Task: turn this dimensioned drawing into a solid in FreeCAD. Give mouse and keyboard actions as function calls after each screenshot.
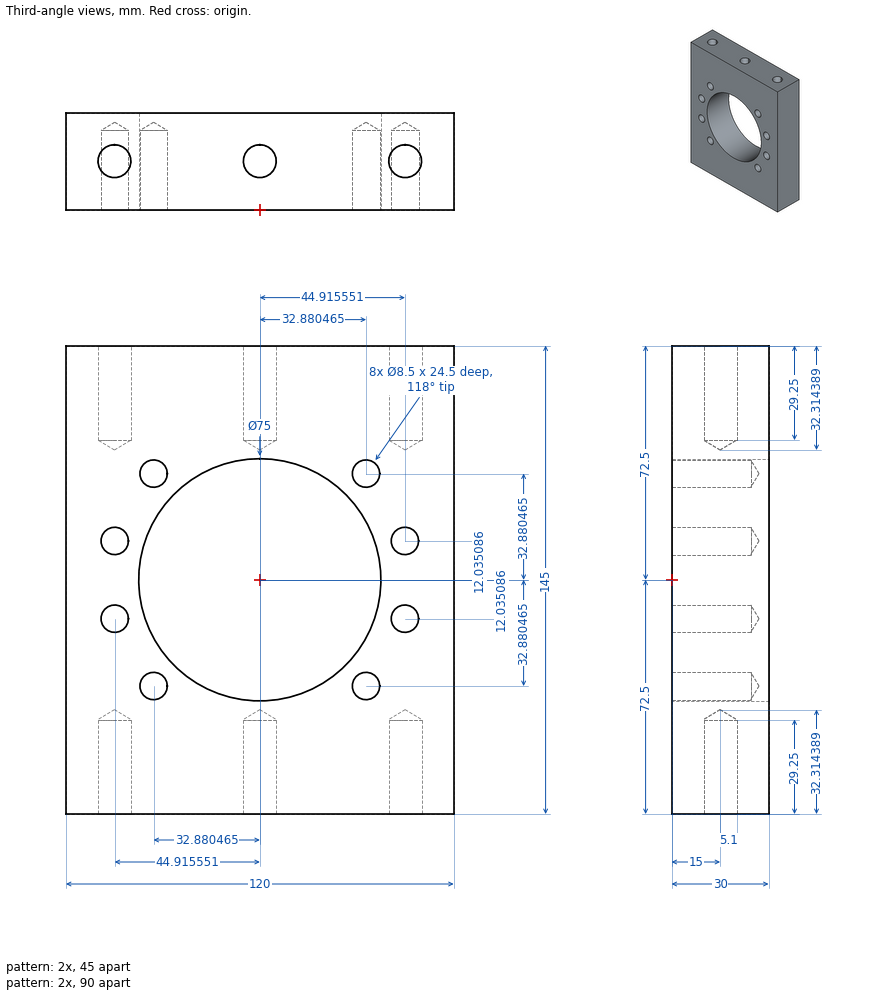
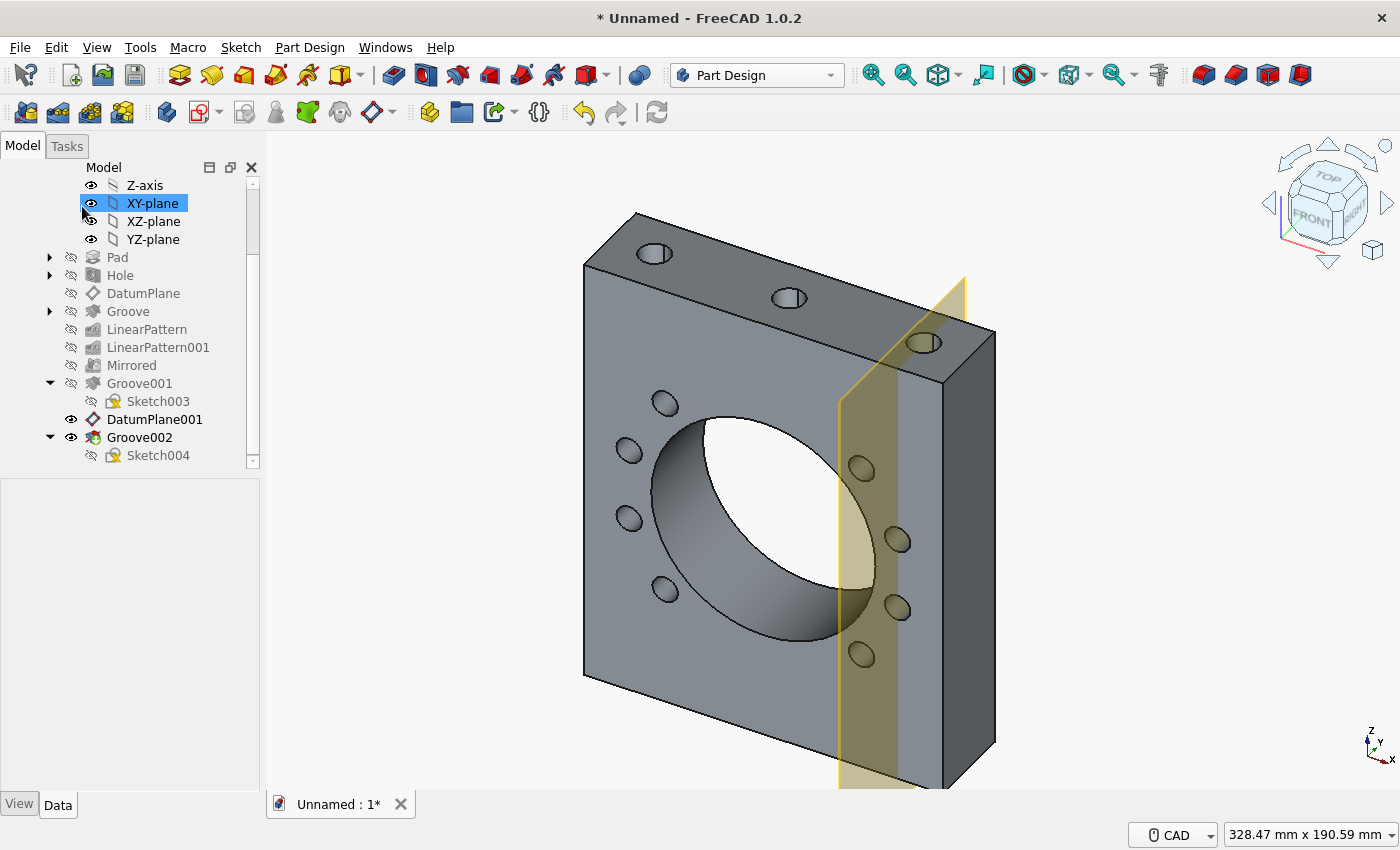
click(116, 419)
key(space)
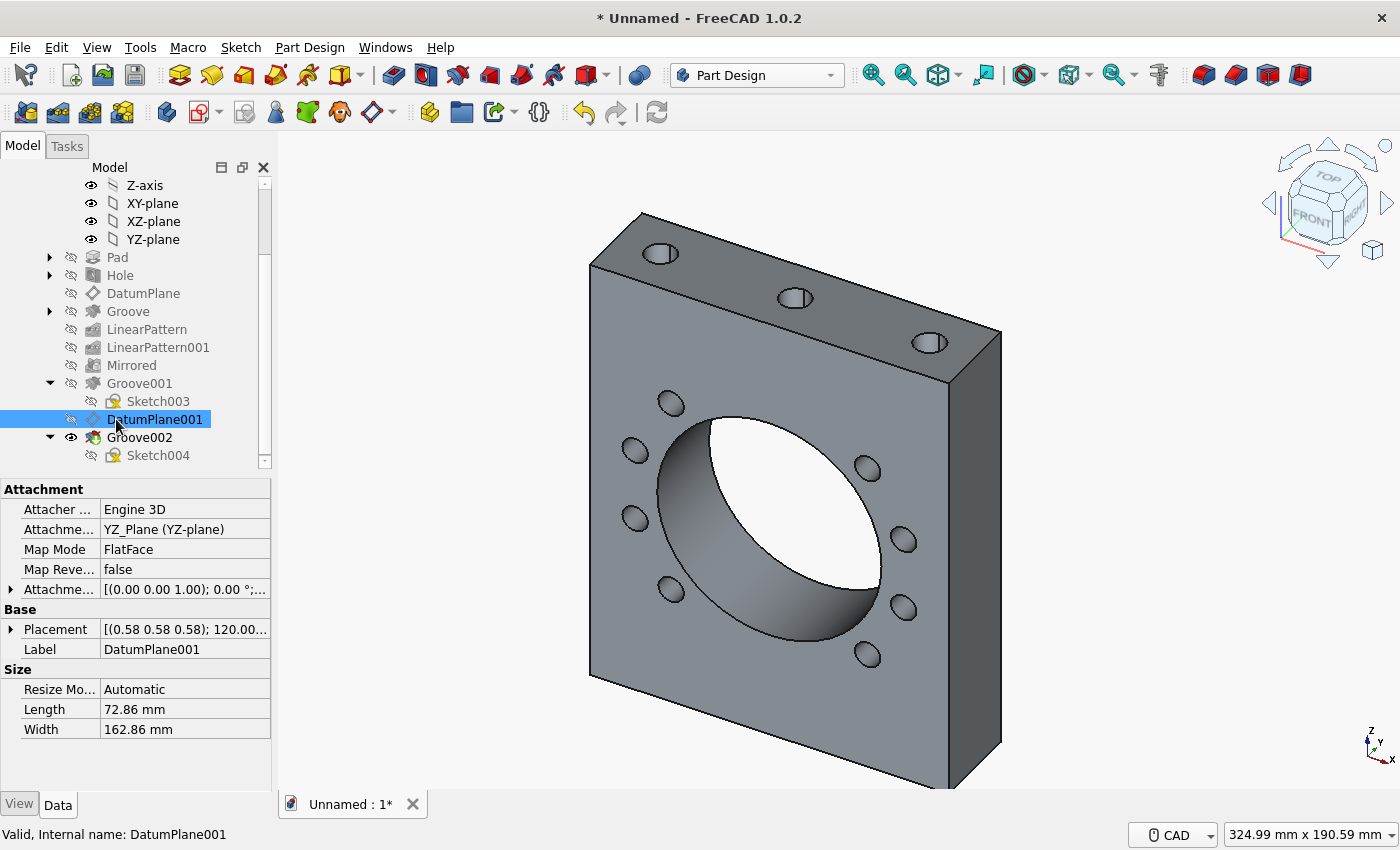
key(0)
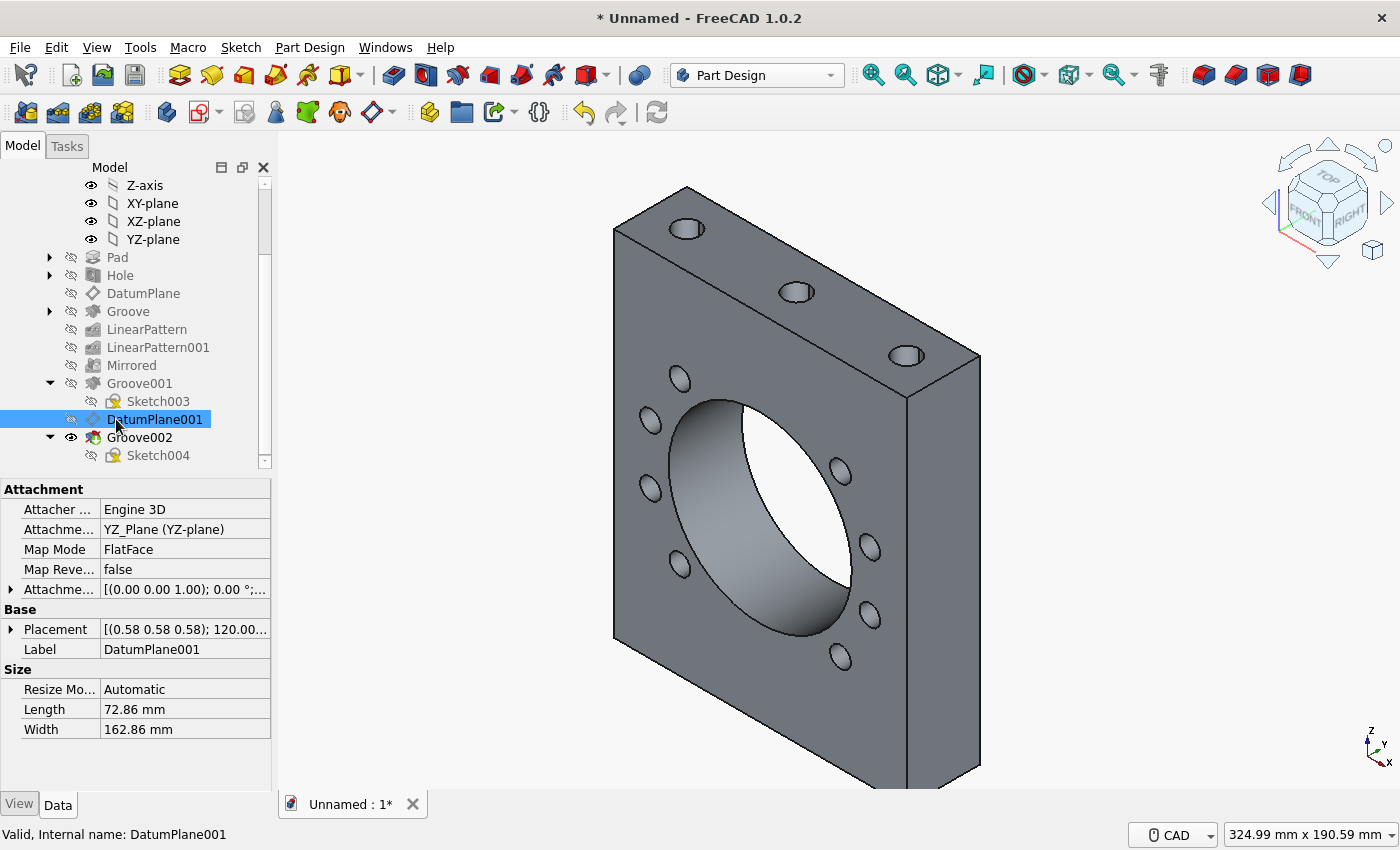
click(874, 76)